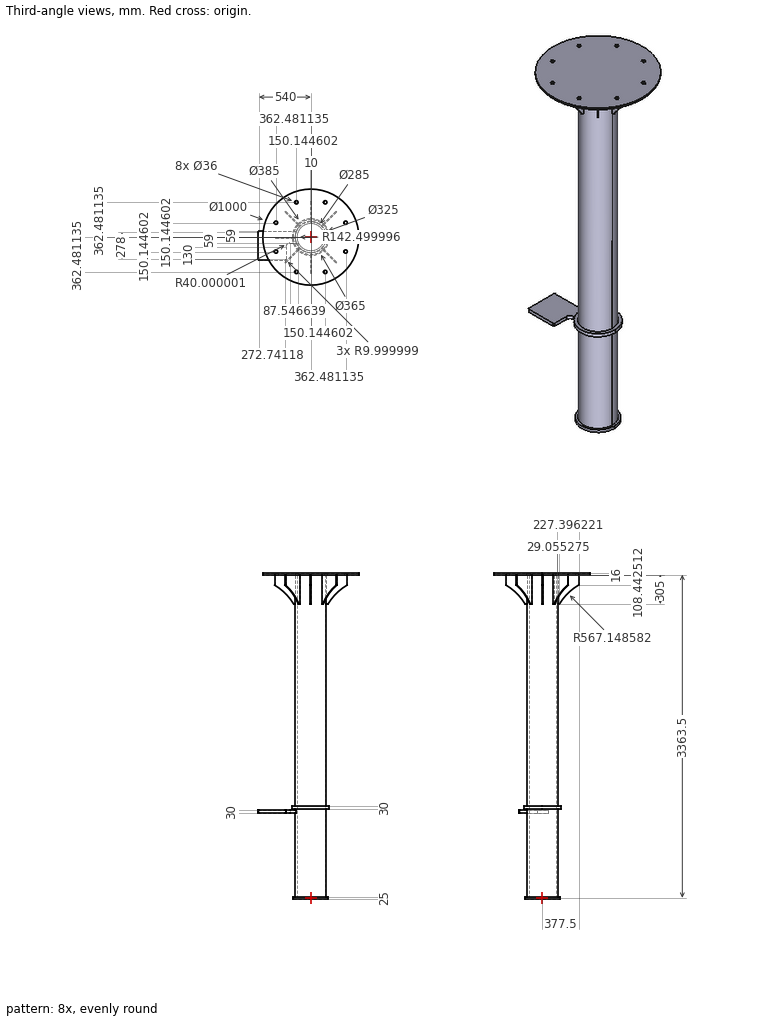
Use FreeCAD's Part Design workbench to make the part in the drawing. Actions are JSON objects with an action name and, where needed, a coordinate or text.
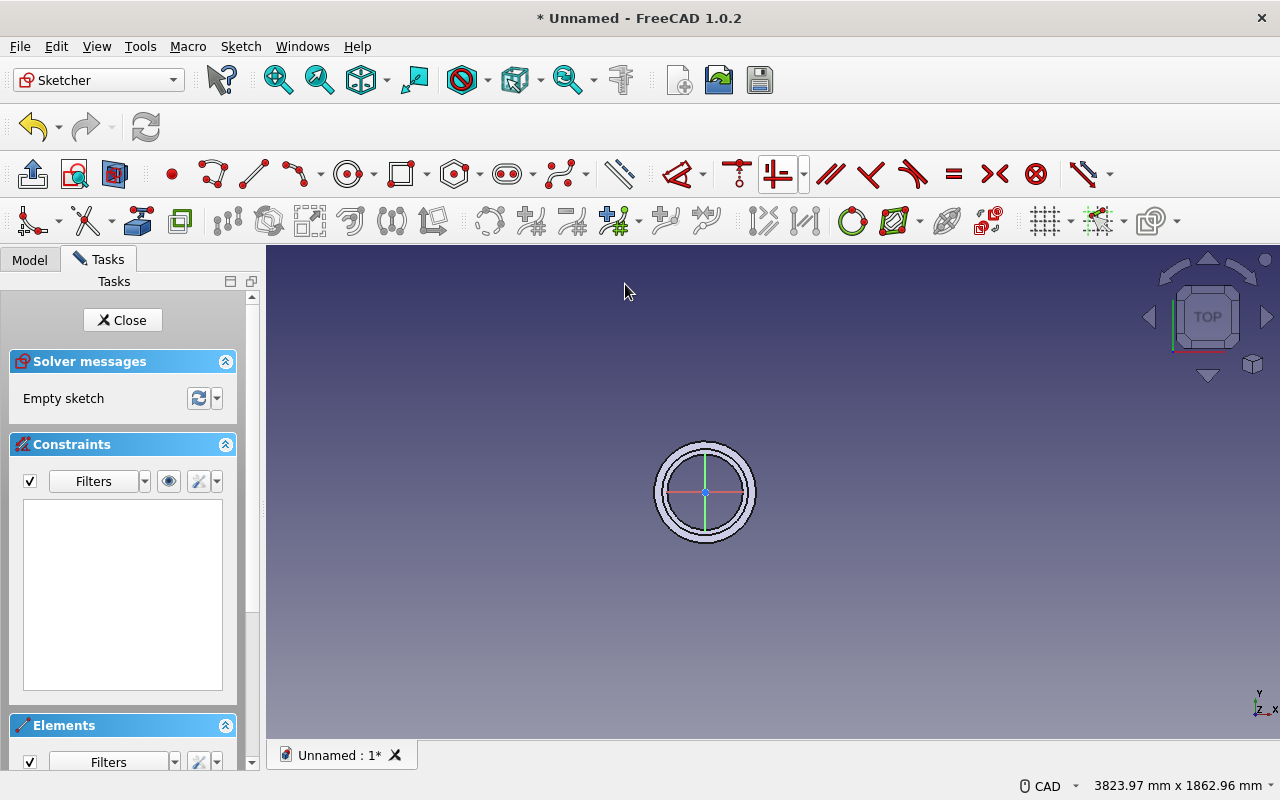
{"action": "key", "text": "g c"}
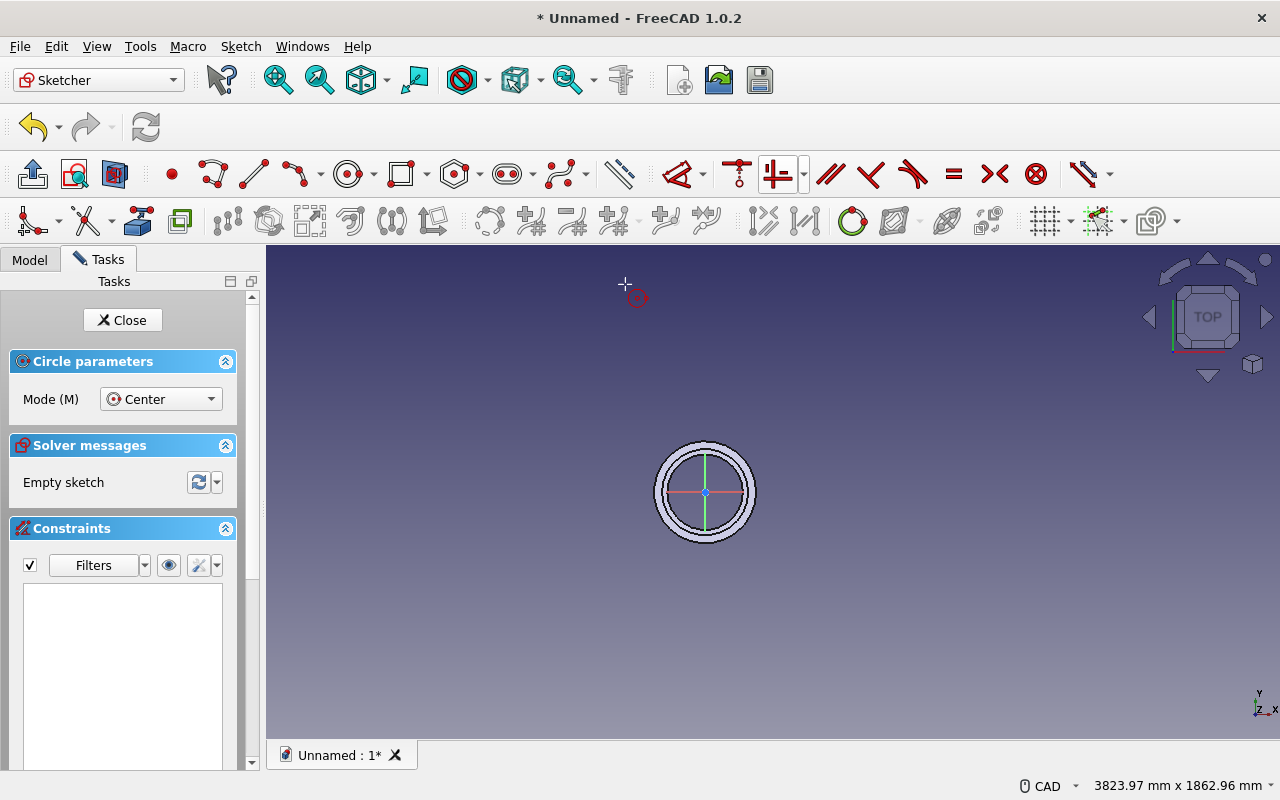
{"action": "left_click", "coordinate": [705, 492]}
{"action": "left_click", "coordinate": [799, 398]}
{"action": "key", "text": "Escape"}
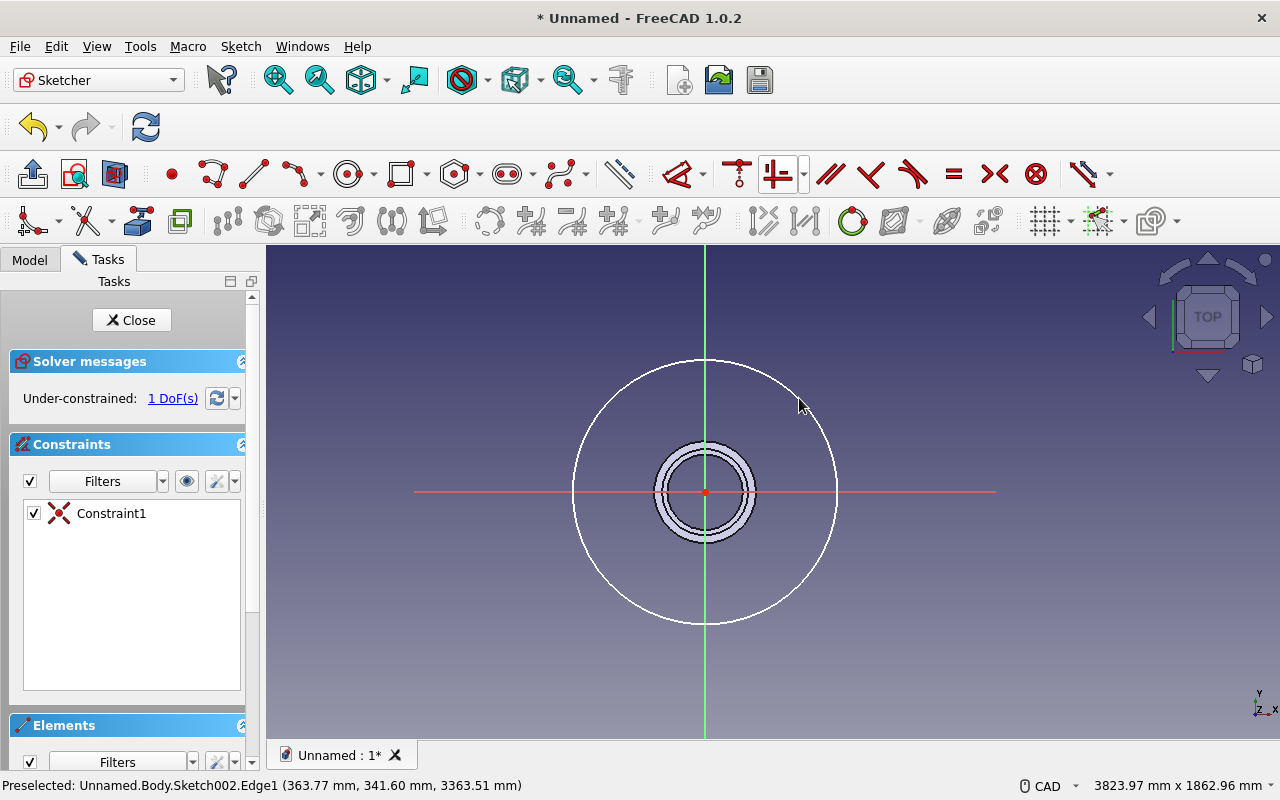
{"action": "left_click", "coordinate": [798, 398]}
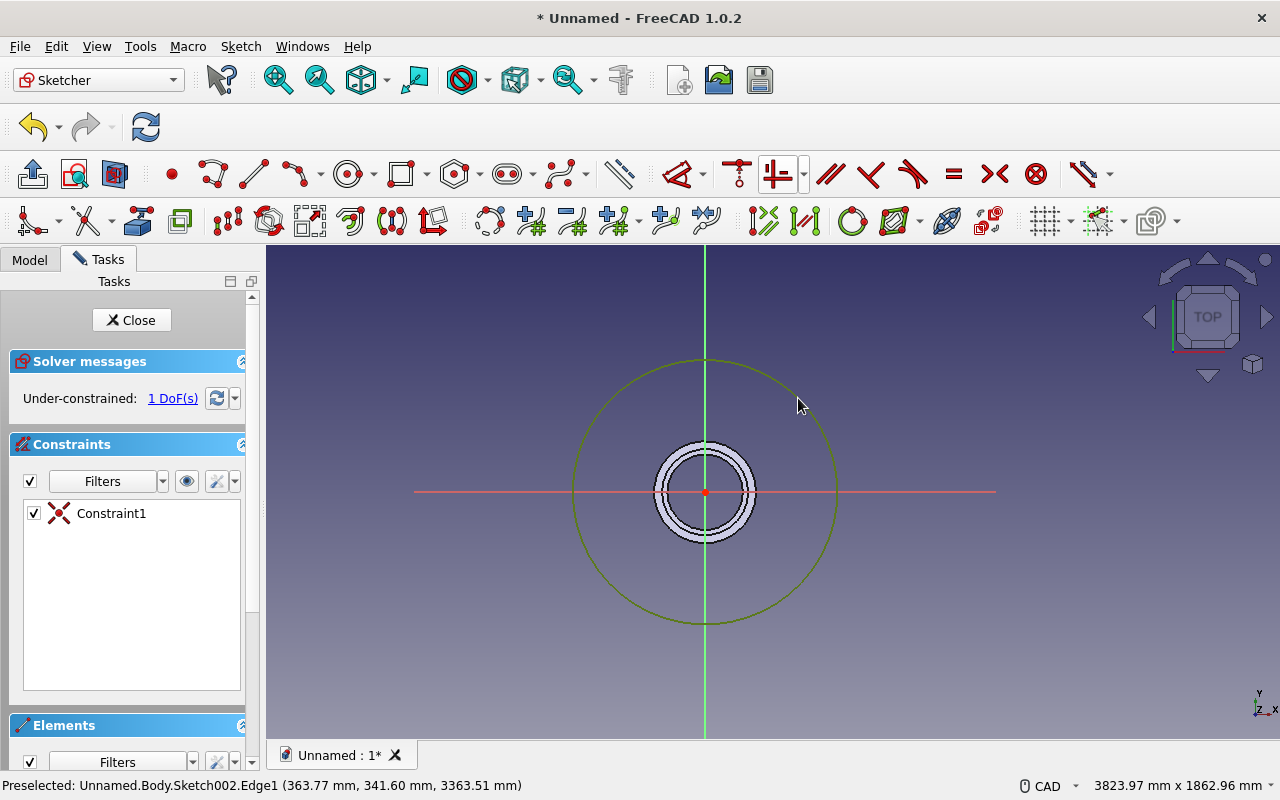
{"action": "left_click", "coordinate": [702, 174]}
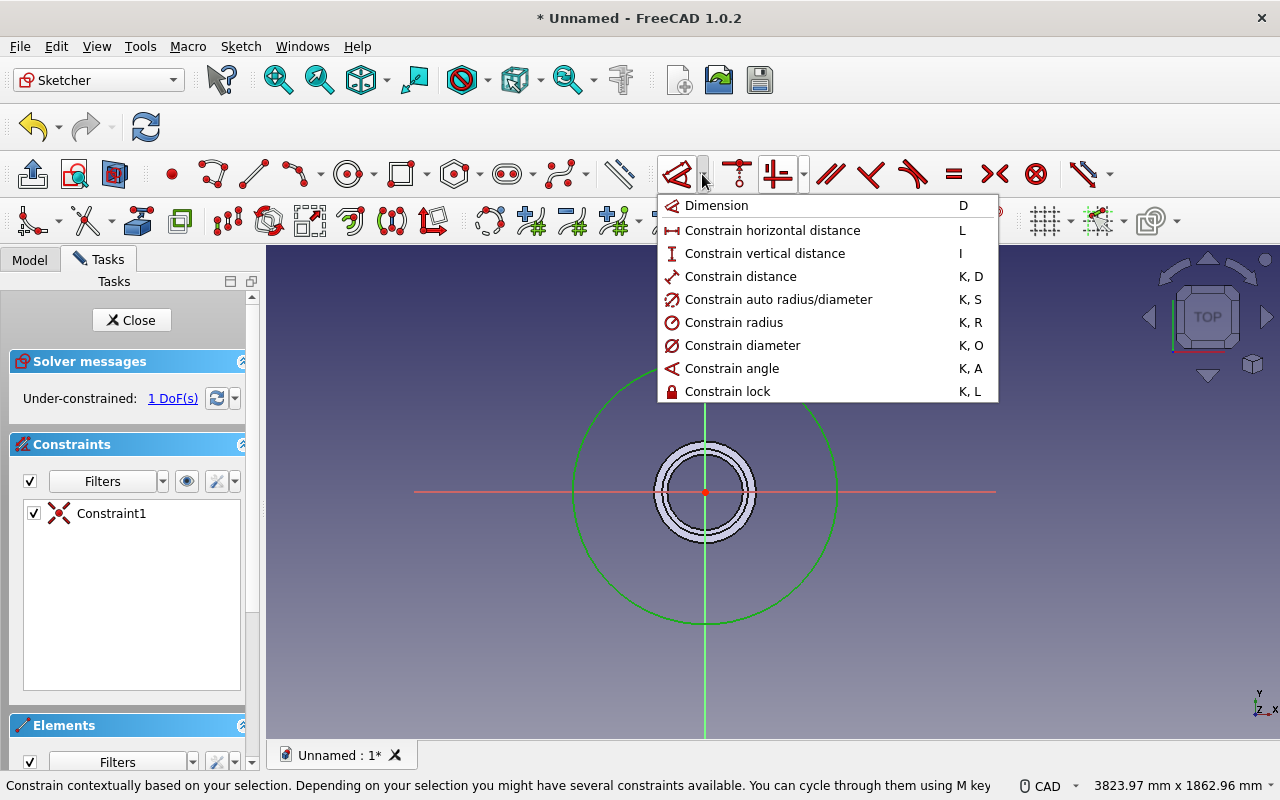
{"action": "left_click", "coordinate": [828, 346]}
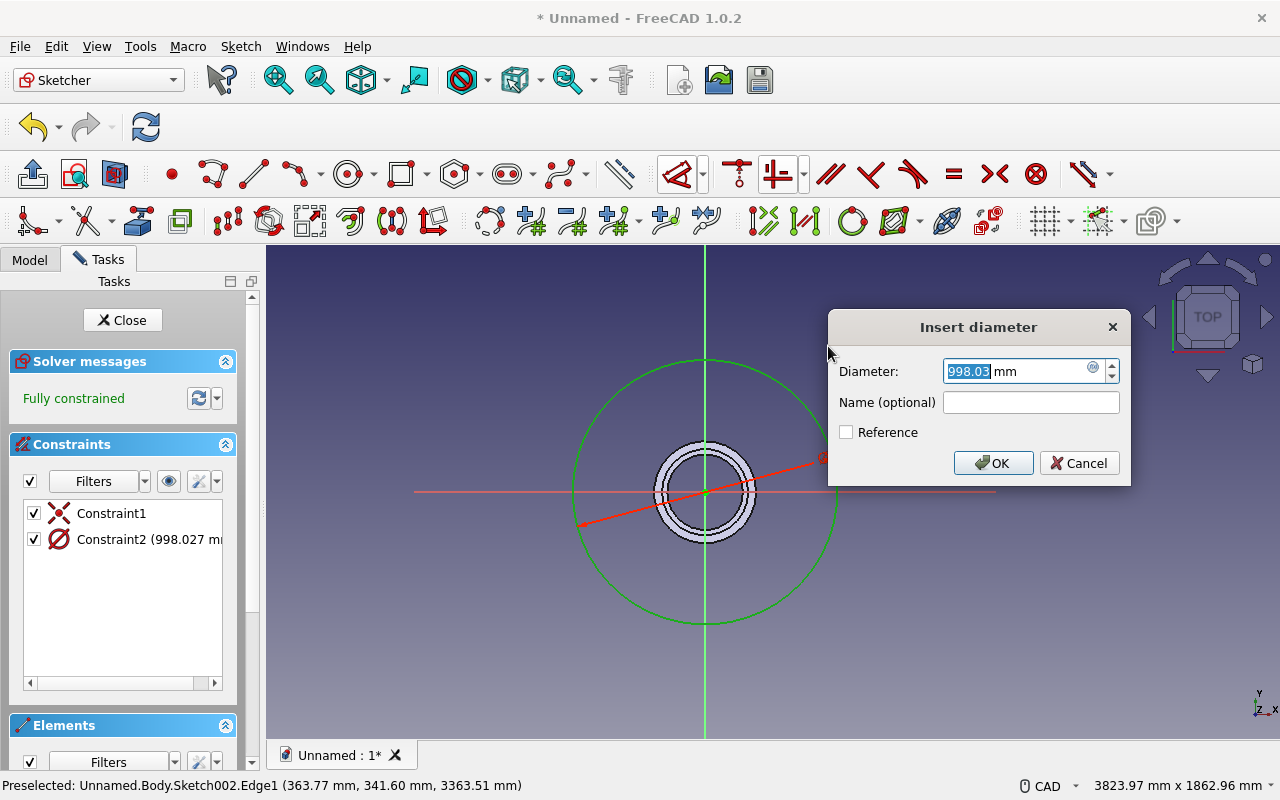
{"action": "type", "text": "1000"}
{"action": "key", "text": "Return"}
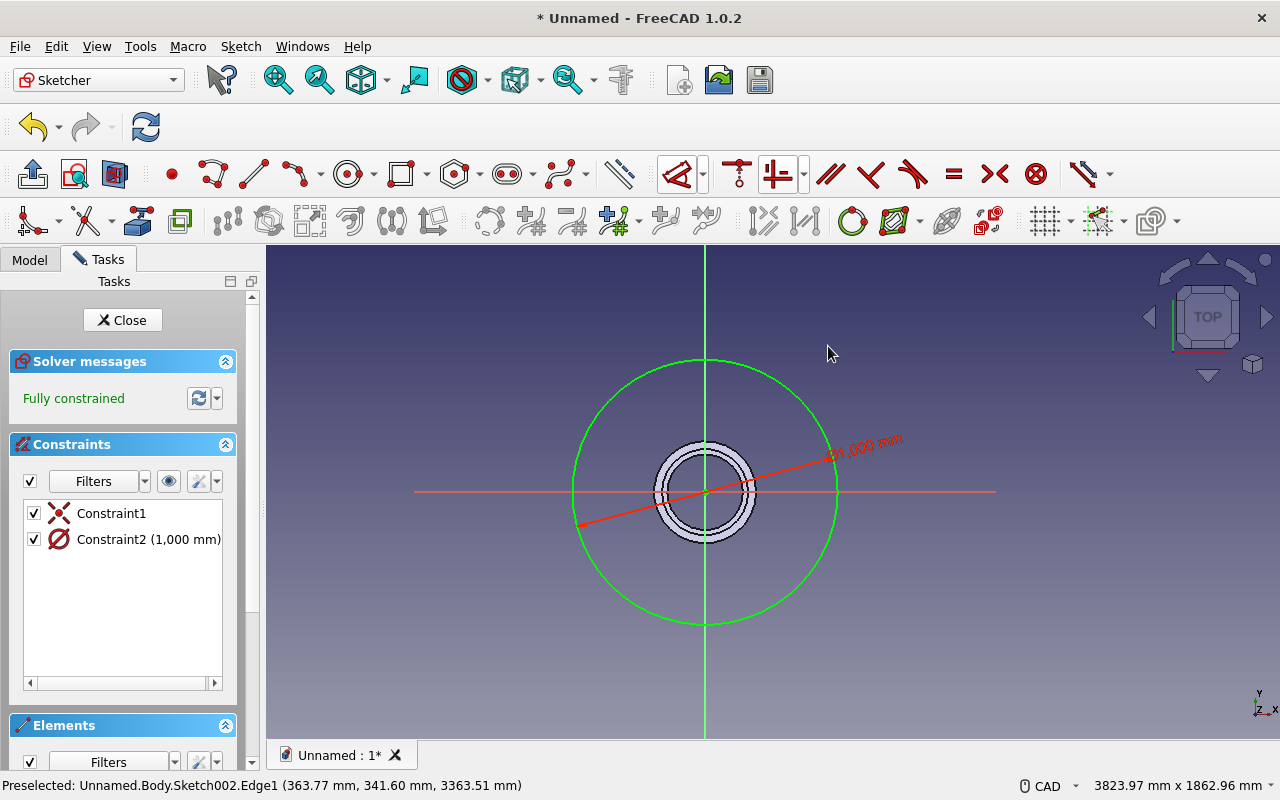
{"action": "left_click", "coordinate": [123, 320]}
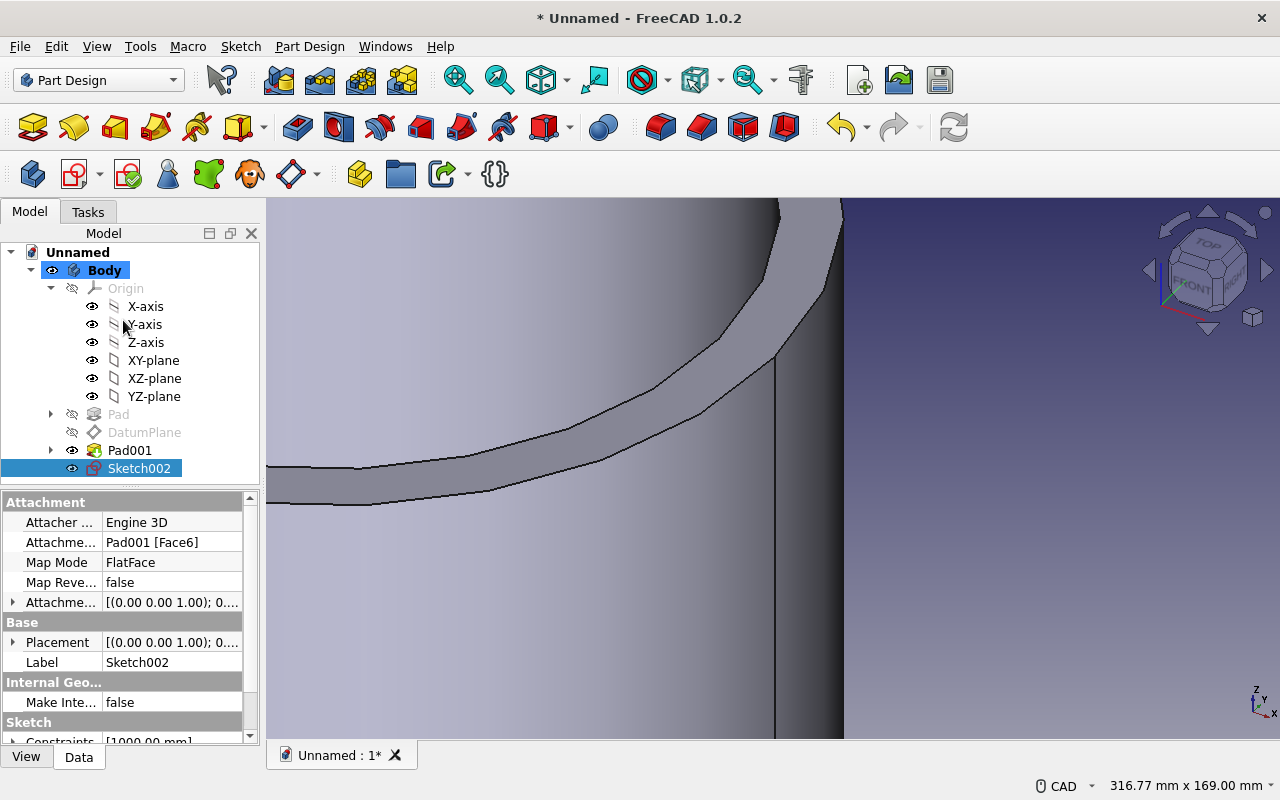
{"action": "left_click", "coordinate": [33, 128]}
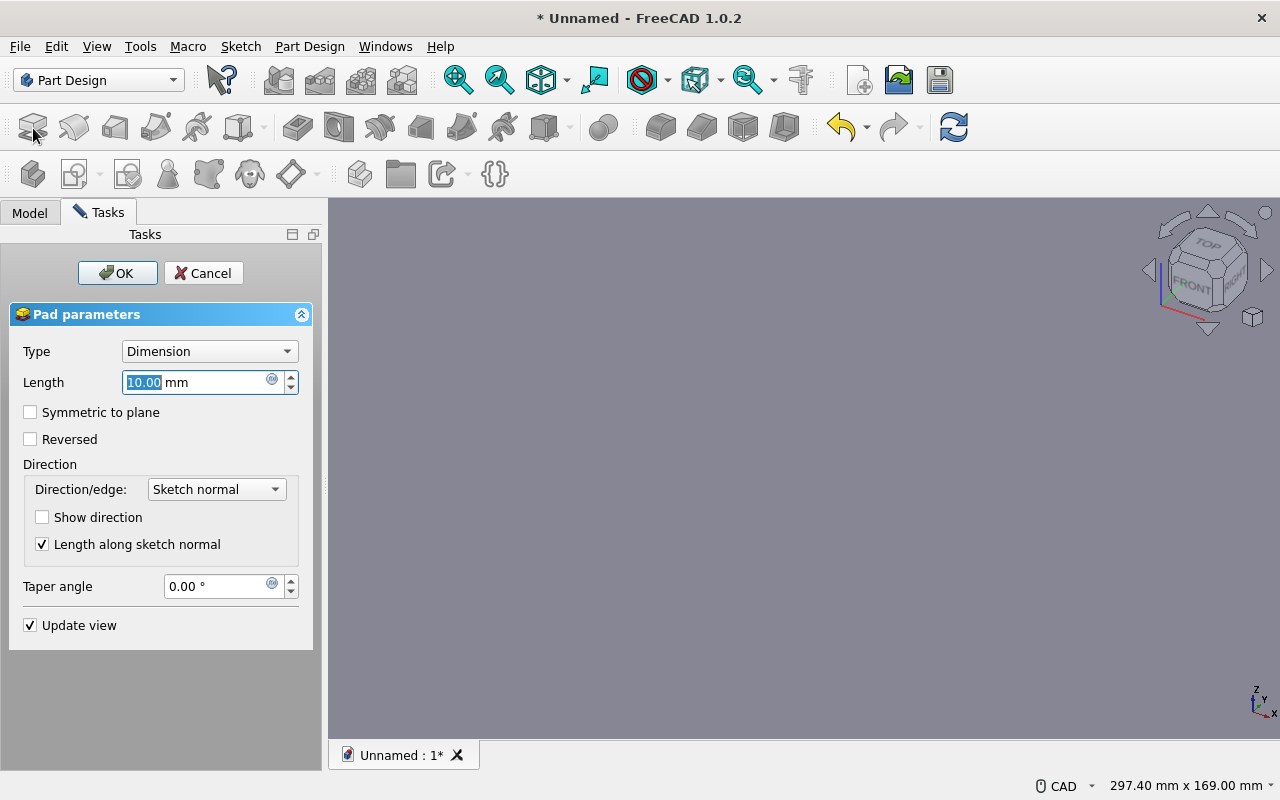
{"action": "type", "text": "16"}
{"action": "key", "text": "Tab"}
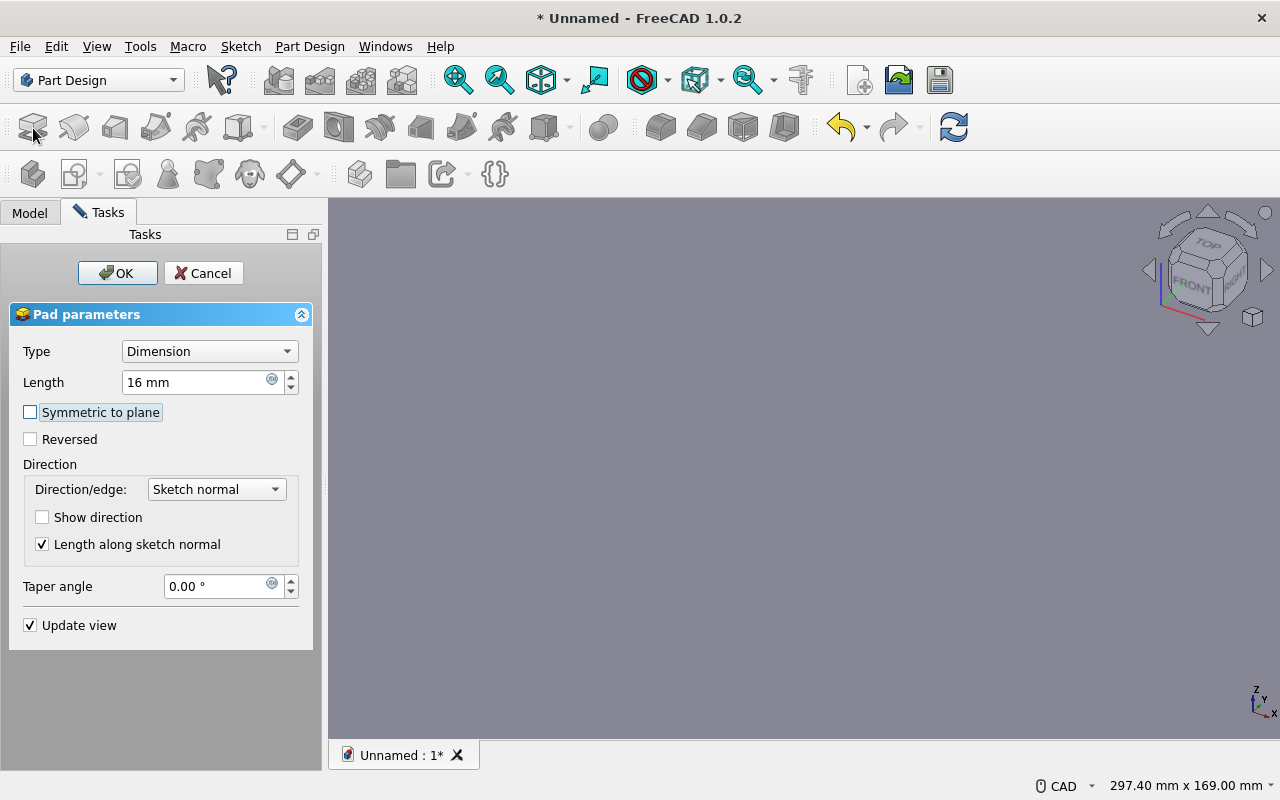
{"action": "left_click", "coordinate": [118, 273]}